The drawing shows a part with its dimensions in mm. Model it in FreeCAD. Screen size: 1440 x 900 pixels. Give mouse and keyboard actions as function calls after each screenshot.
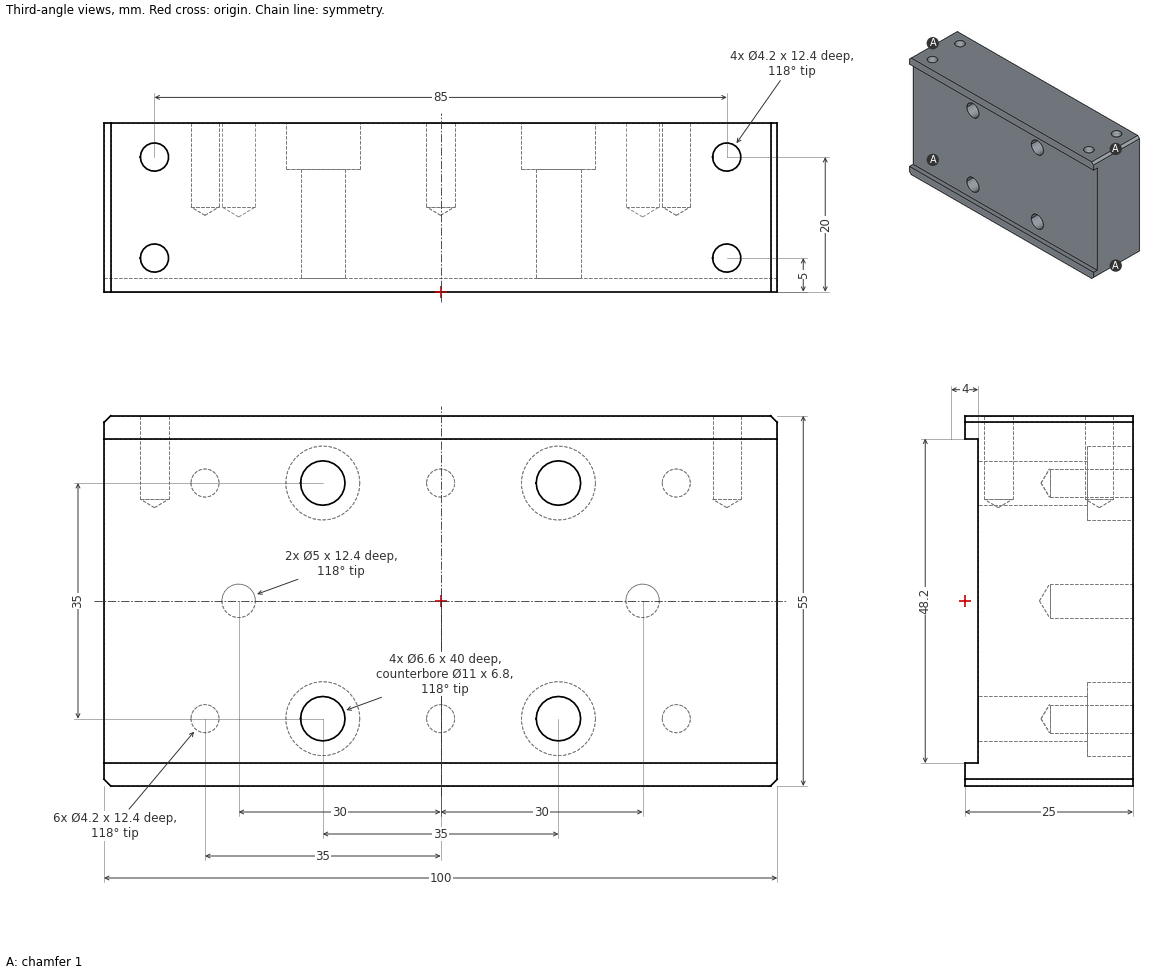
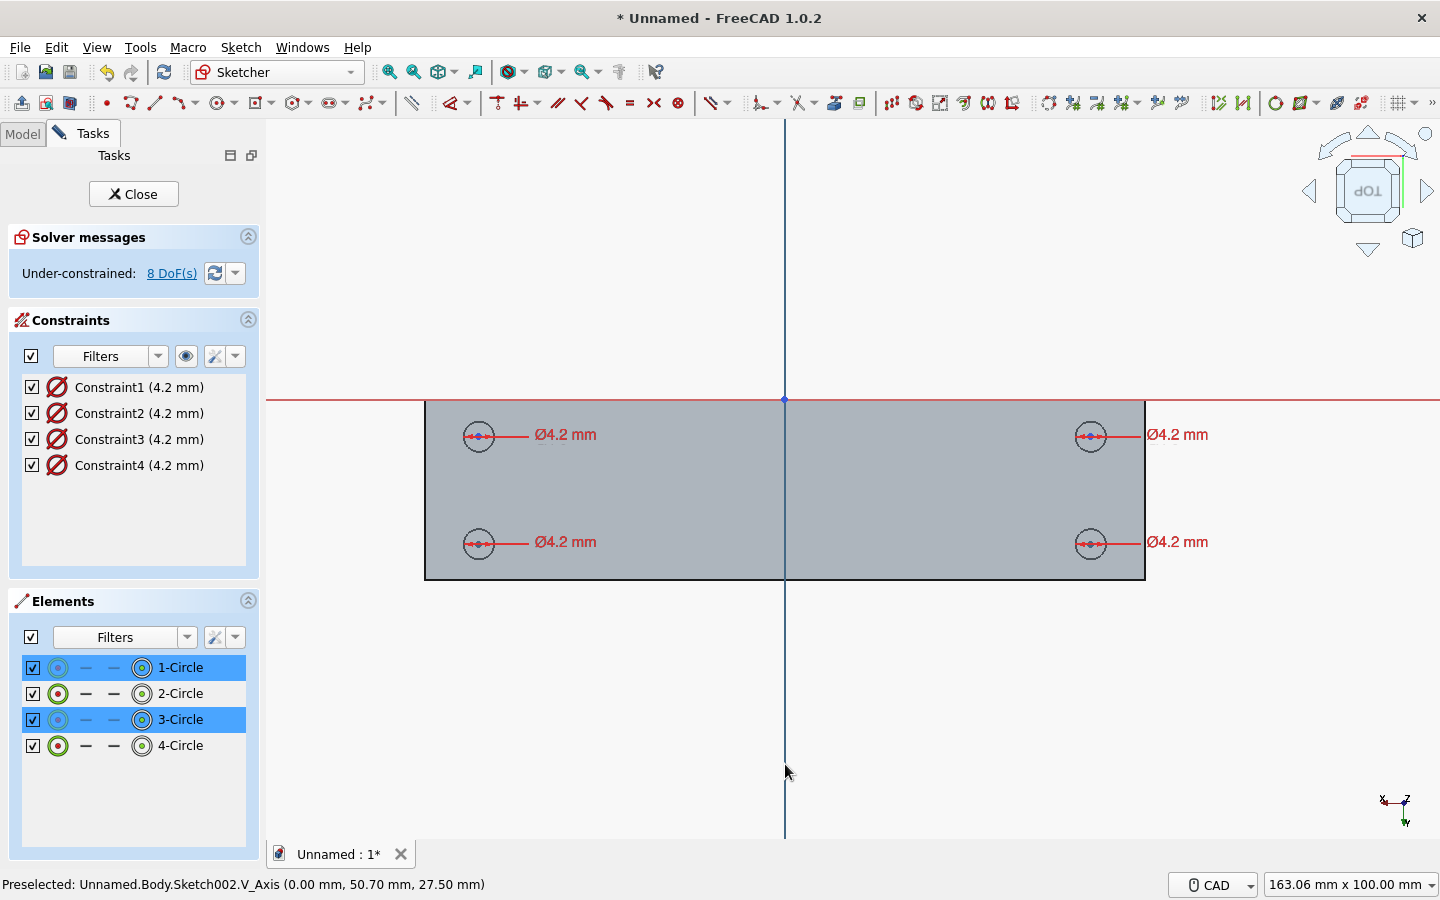
click(654, 104)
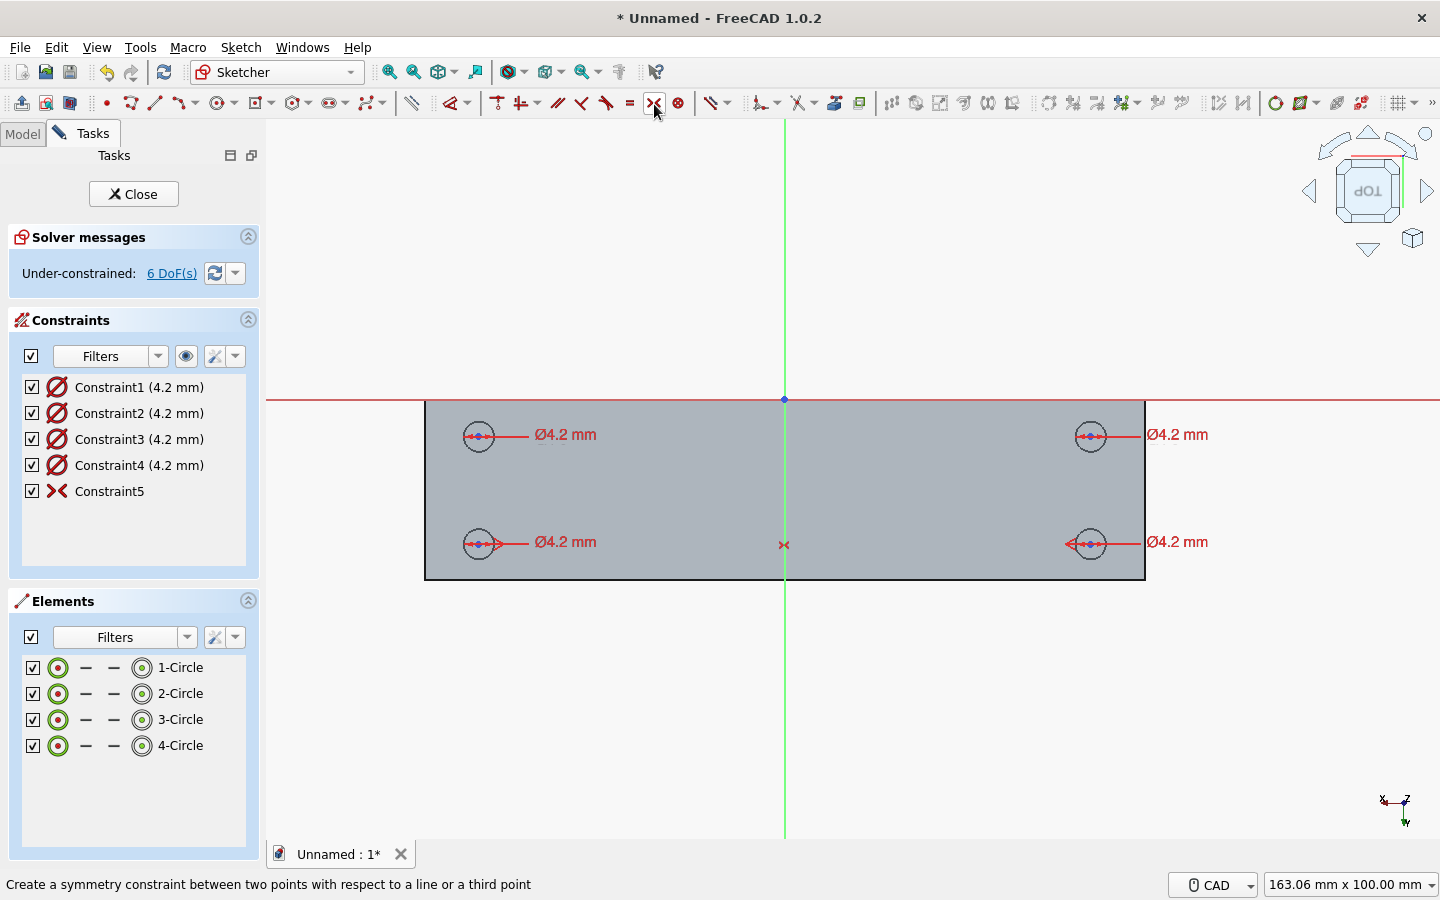
click(479, 437)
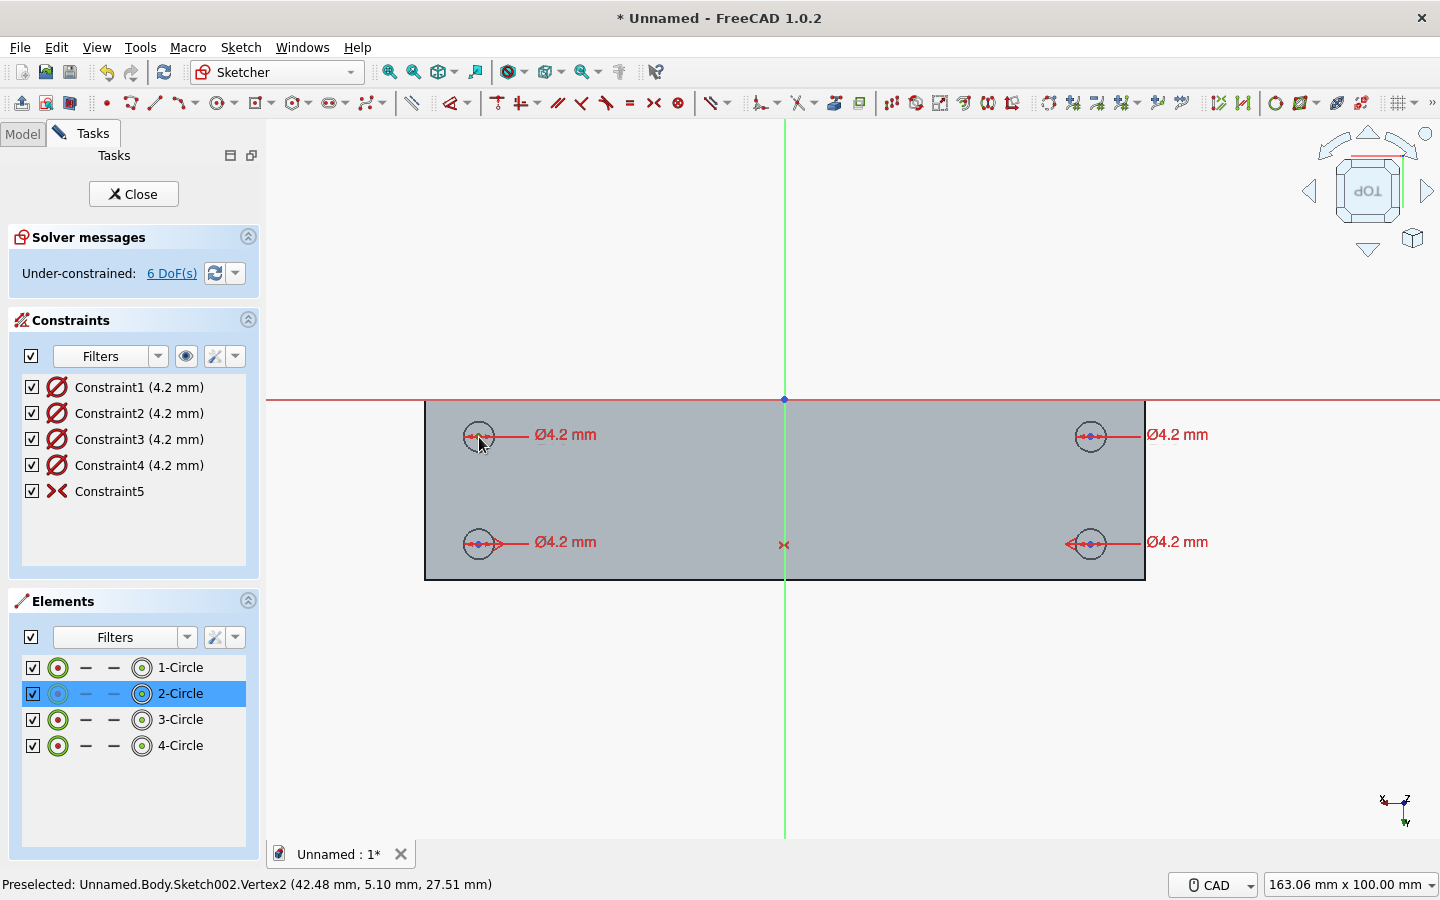
click(1091, 437)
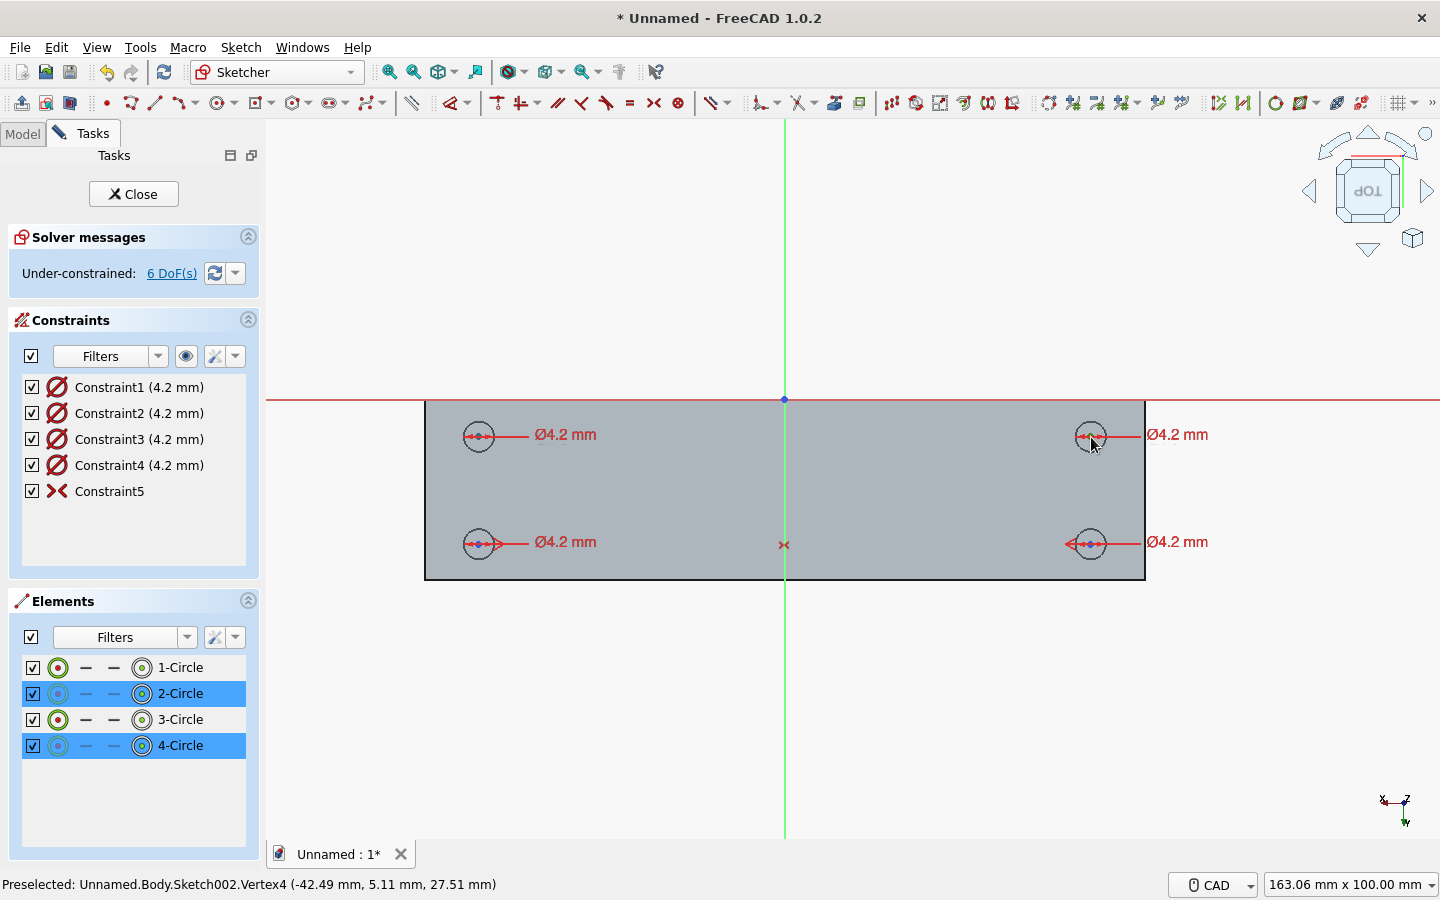
click(785, 764)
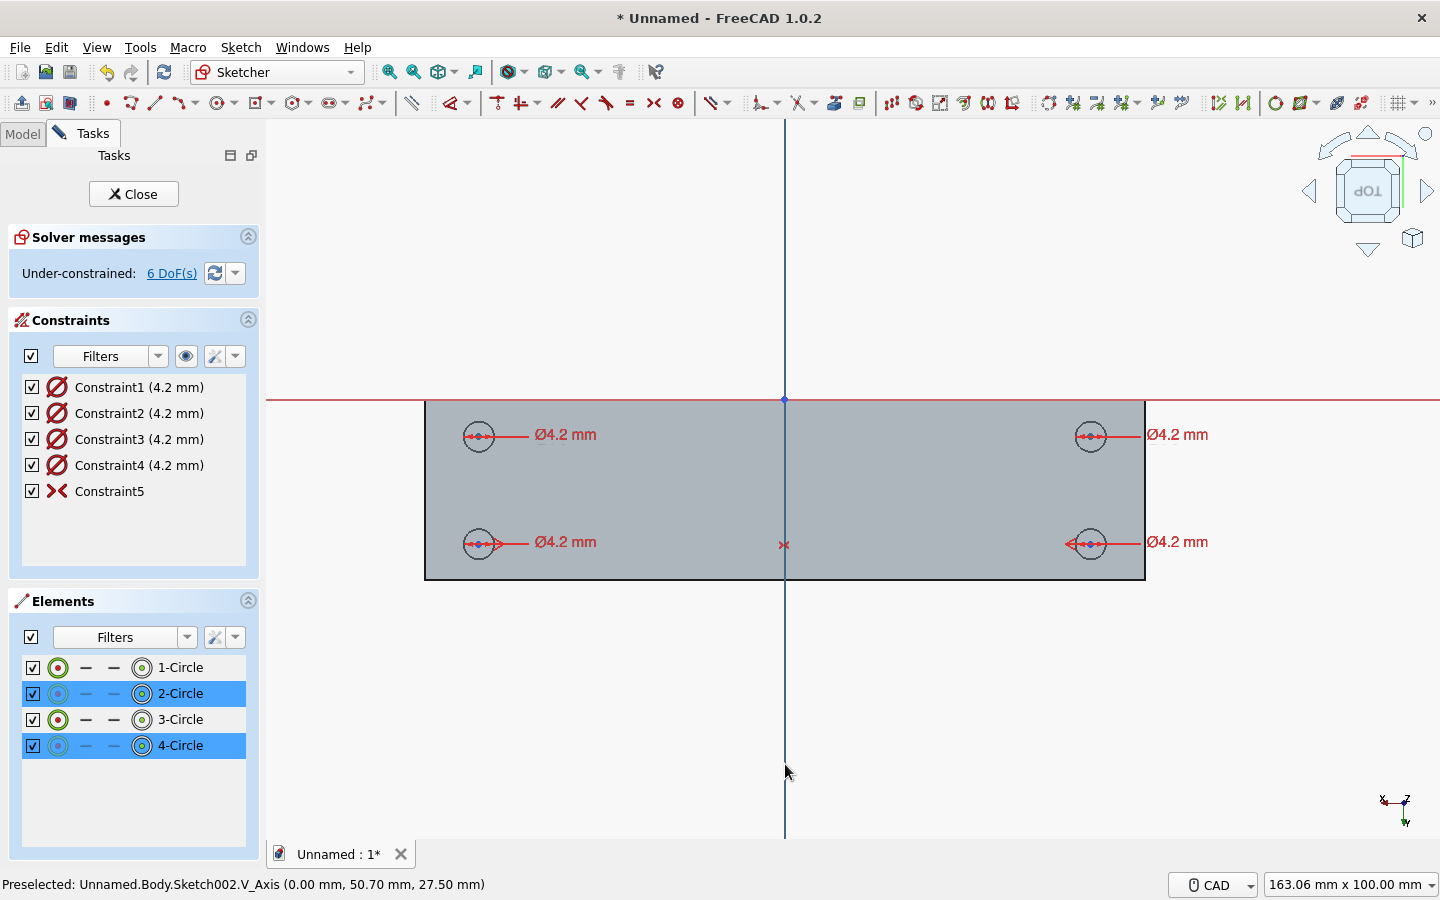
click(654, 104)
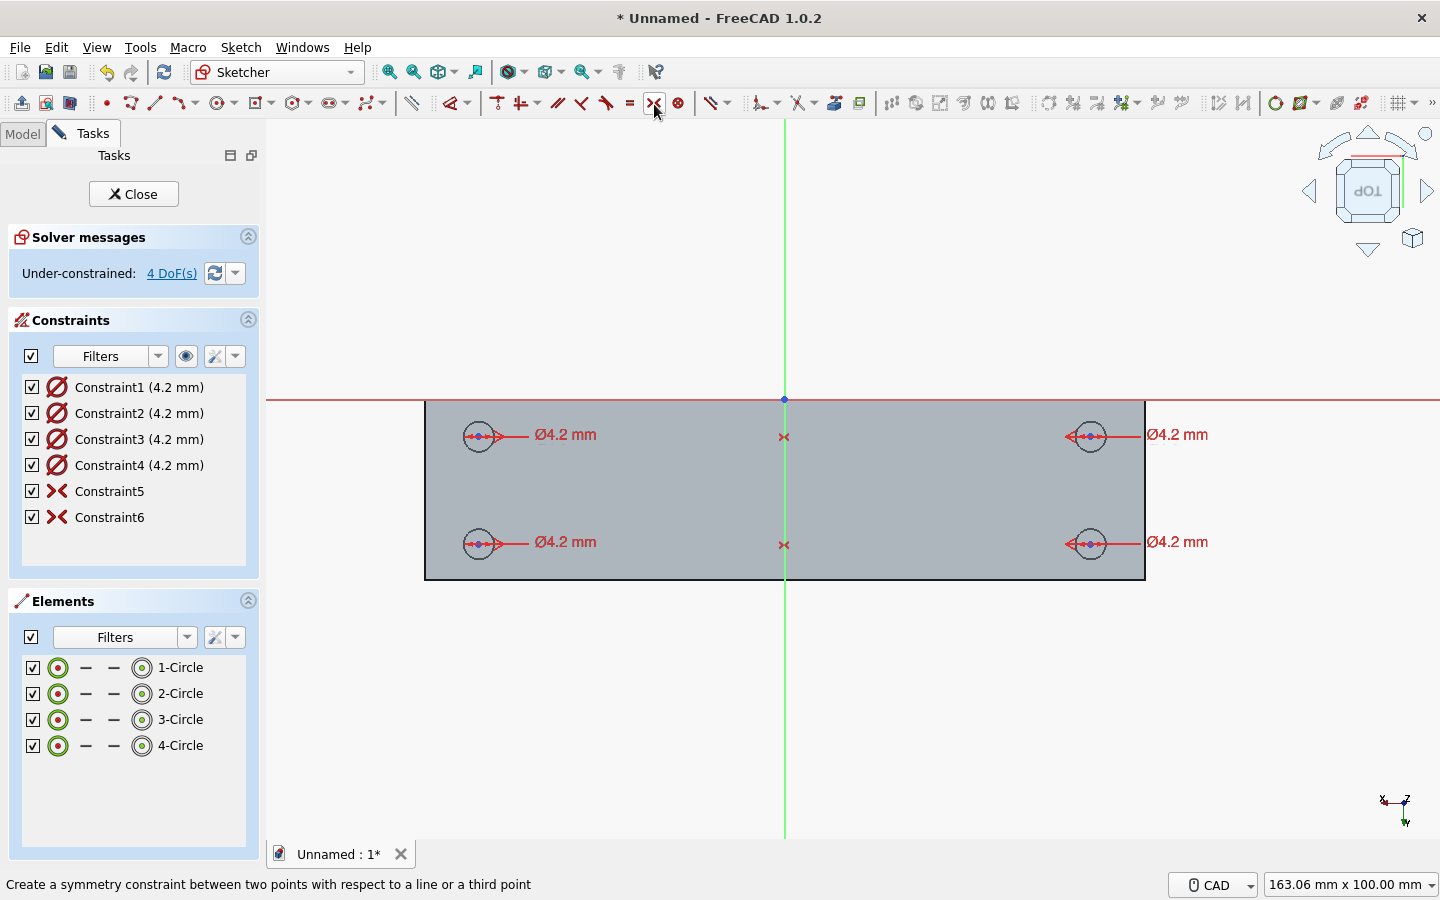
click(450, 104)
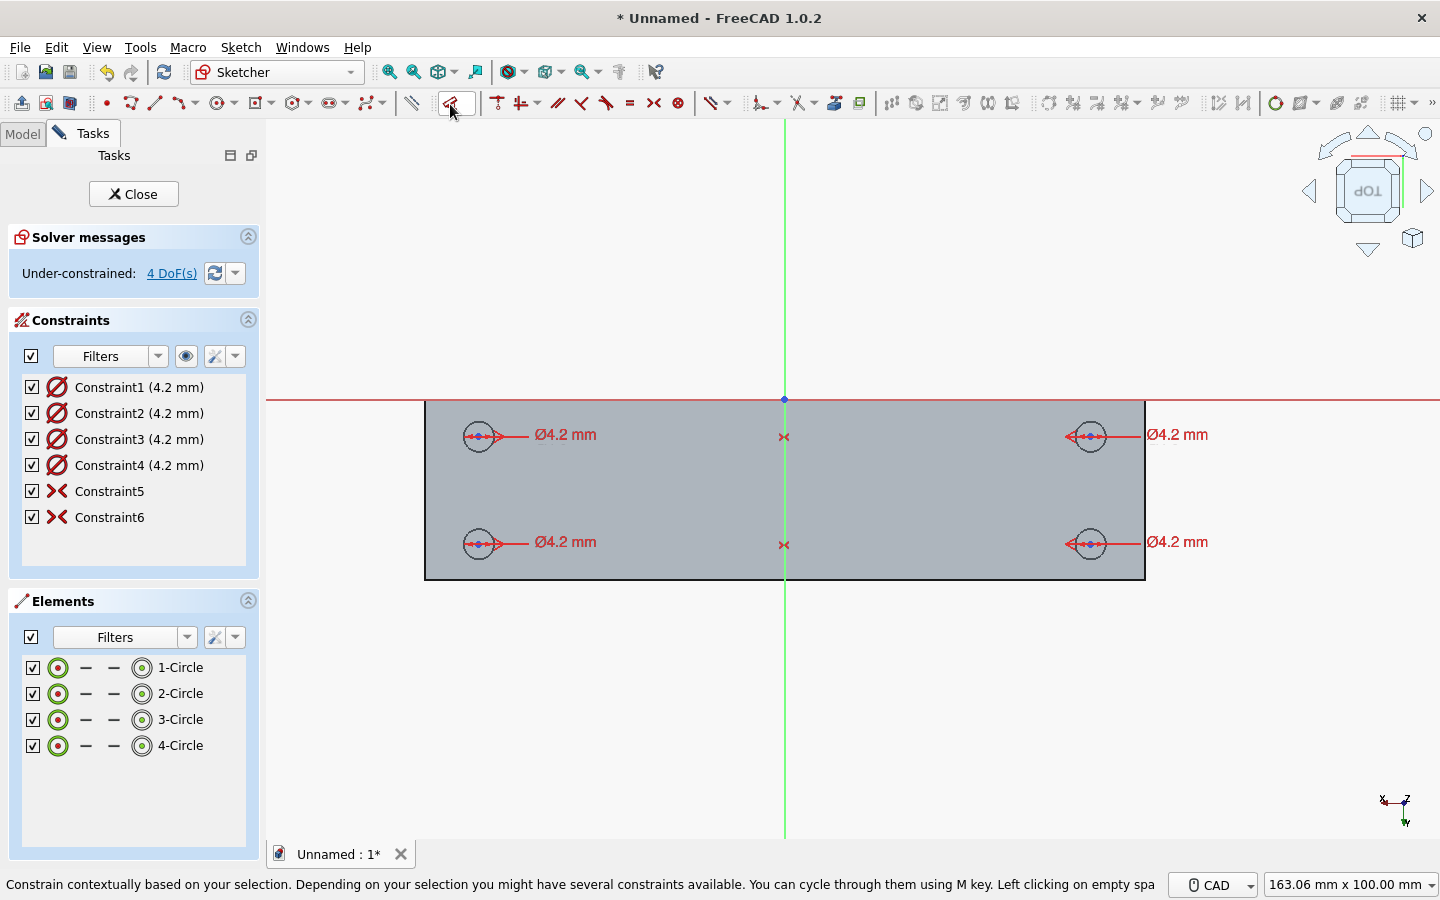
click(479, 437)
click(445, 418)